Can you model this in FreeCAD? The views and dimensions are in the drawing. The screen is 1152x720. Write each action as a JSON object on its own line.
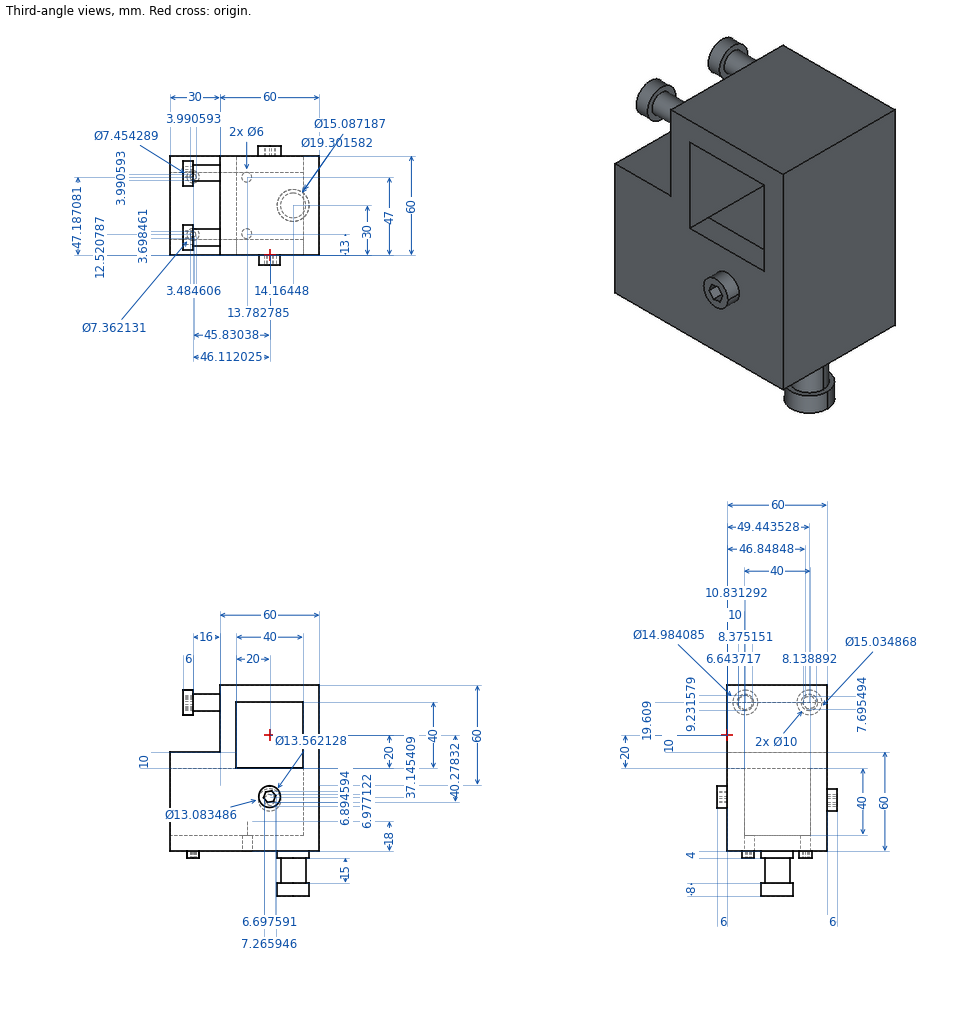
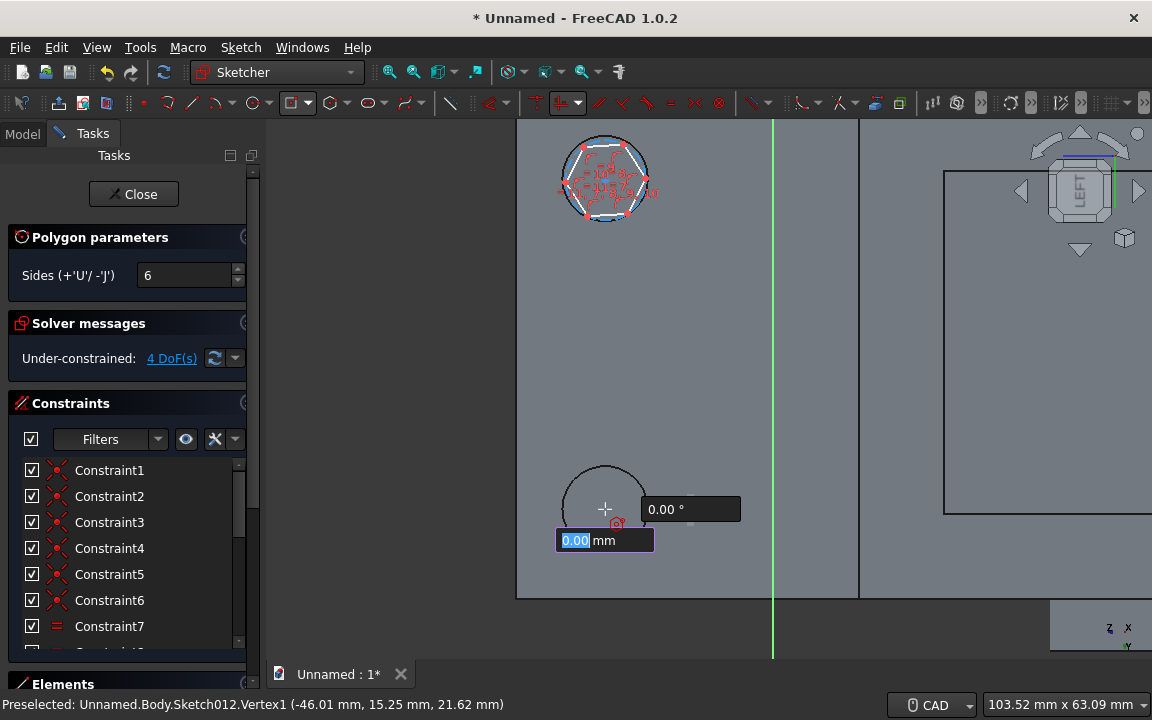
{"action": "left_click", "coordinate": [572, 522]}
{"action": "right_click", "coordinate": [572, 522]}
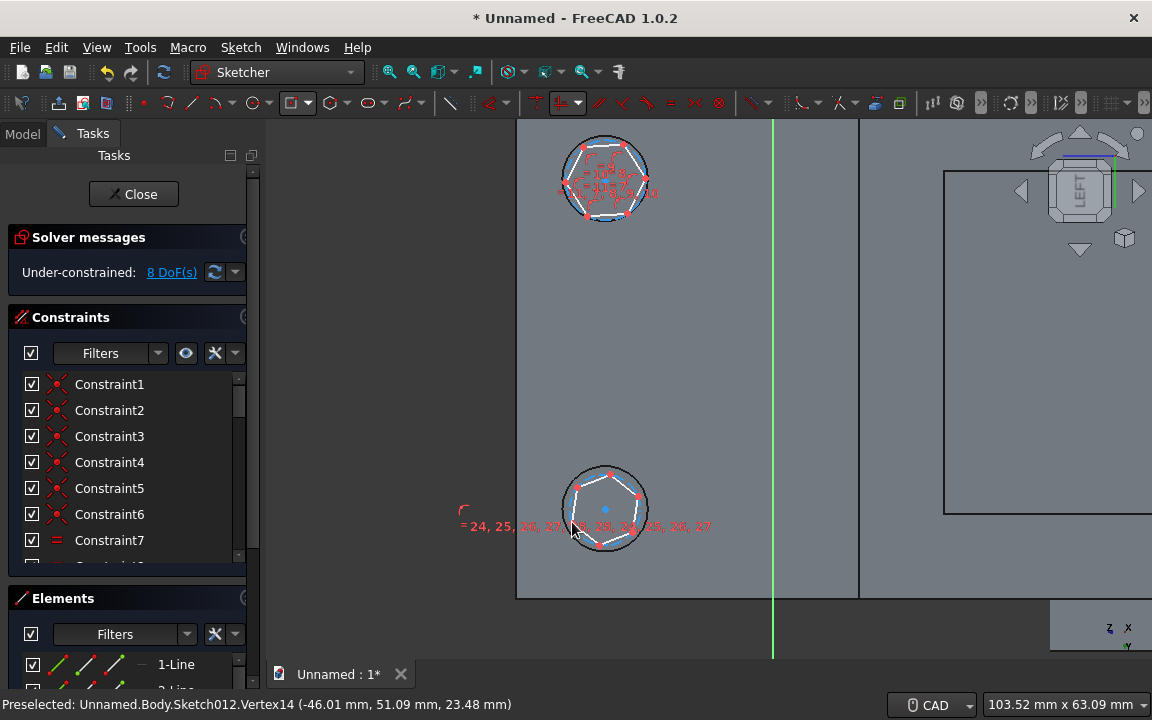
{"action": "left_click", "coordinate": [254, 104]}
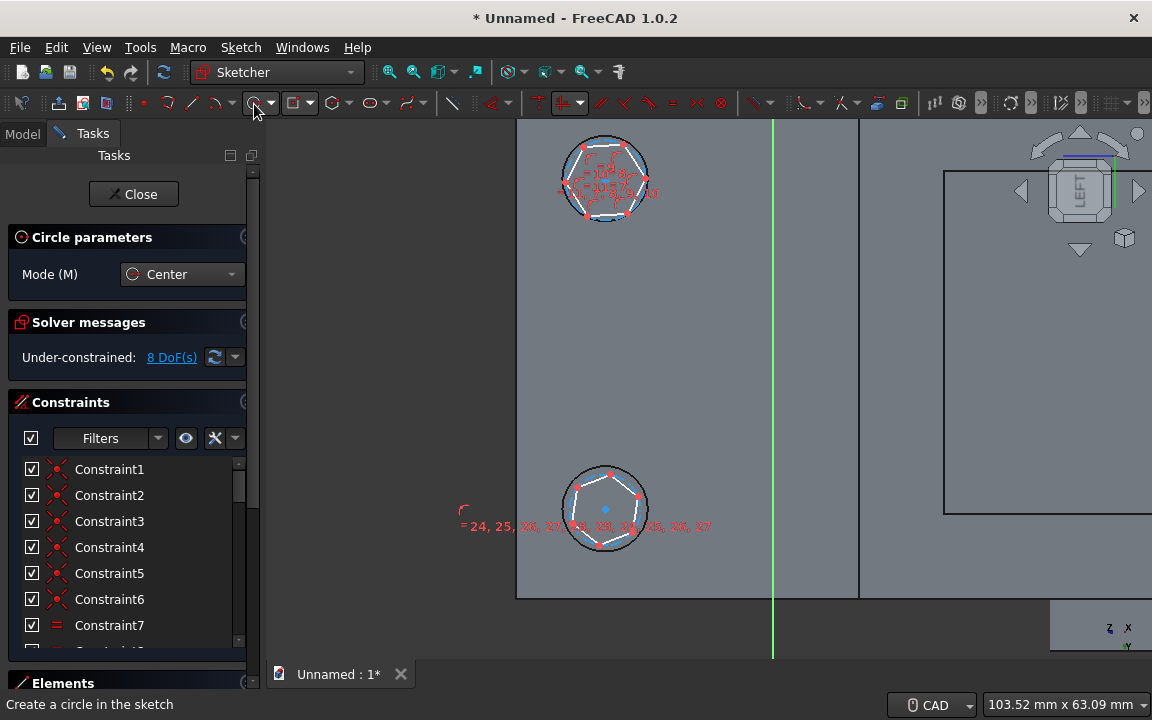
{"action": "left_click", "coordinate": [606, 180]}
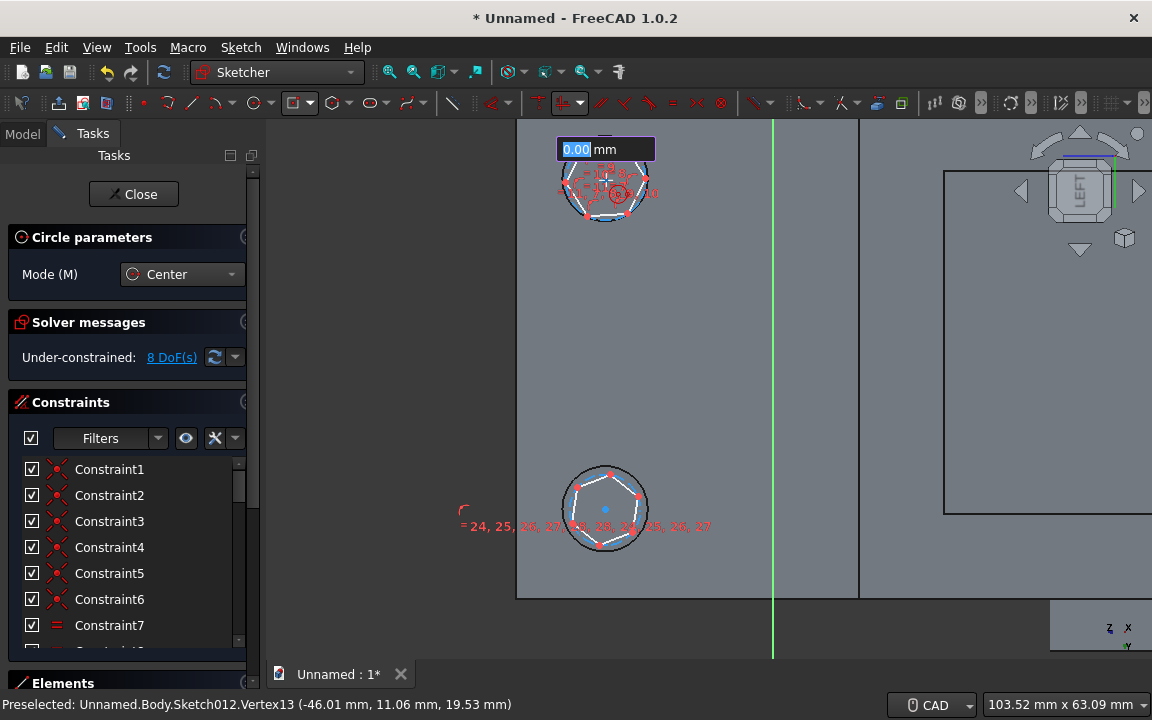
{"action": "scroll", "coordinate": [607, 510], "scroll_direction": "down", "scroll_amount": 2}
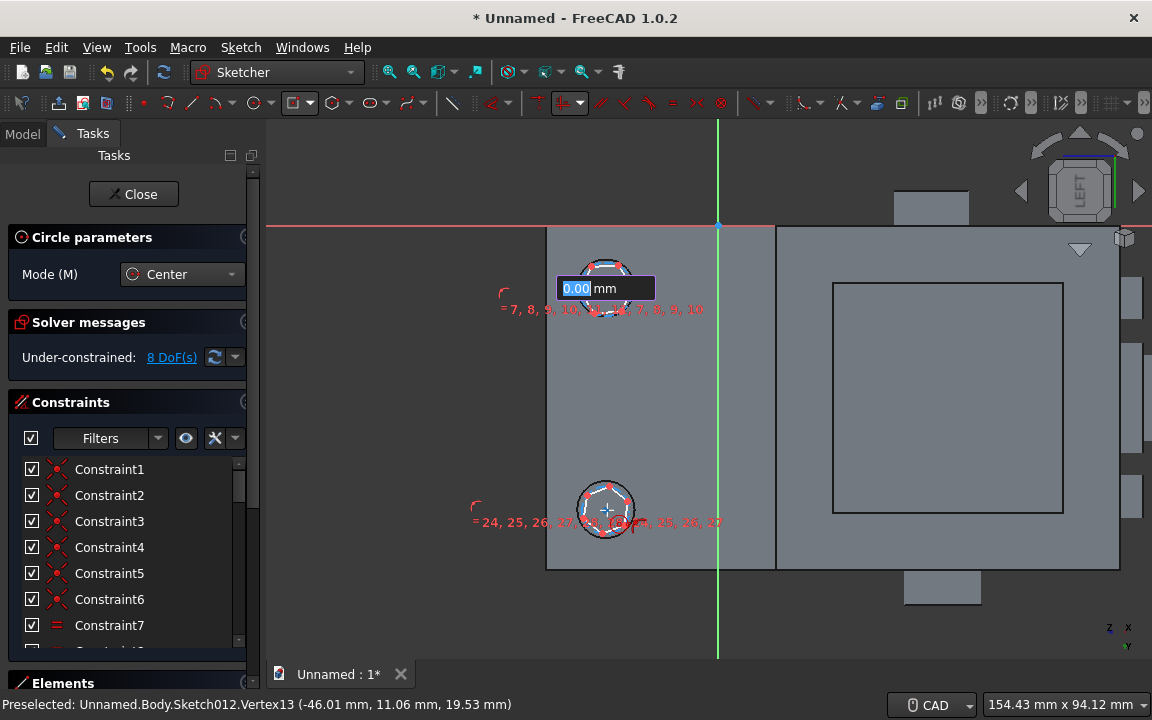
{"action": "left_click", "coordinate": [636, 258]}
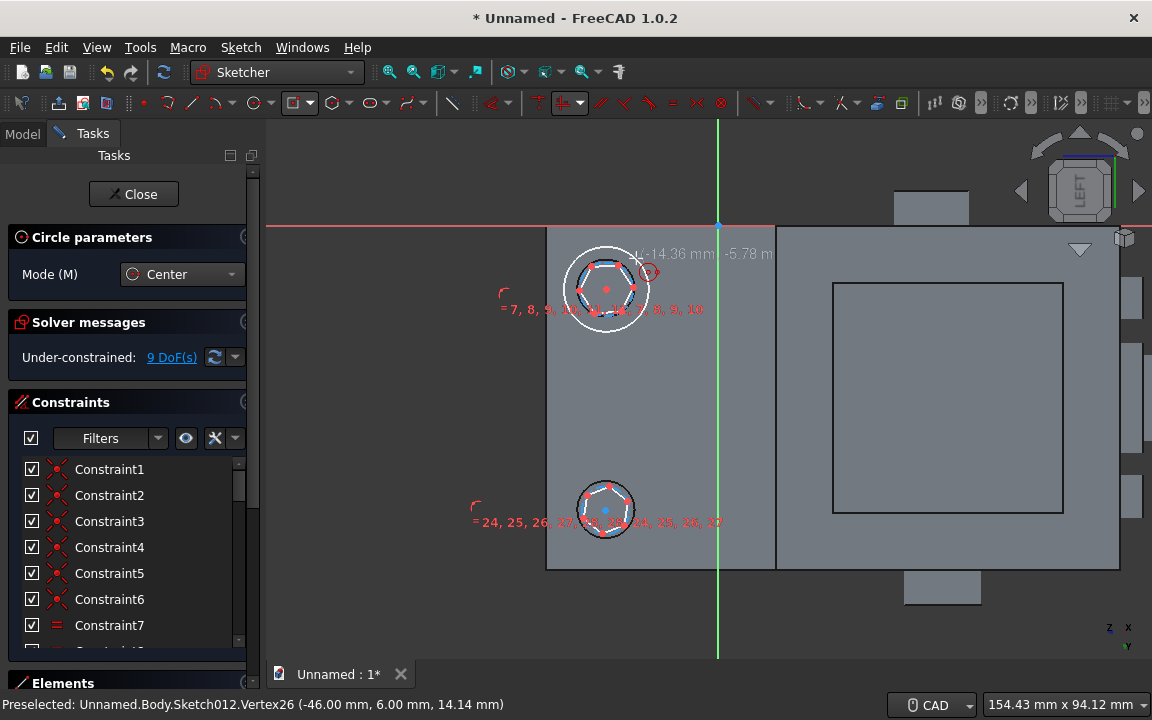
{"action": "left_click", "coordinate": [606, 510]}
{"action": "left_click", "coordinate": [636, 479]}
{"action": "key", "text": "Escape"}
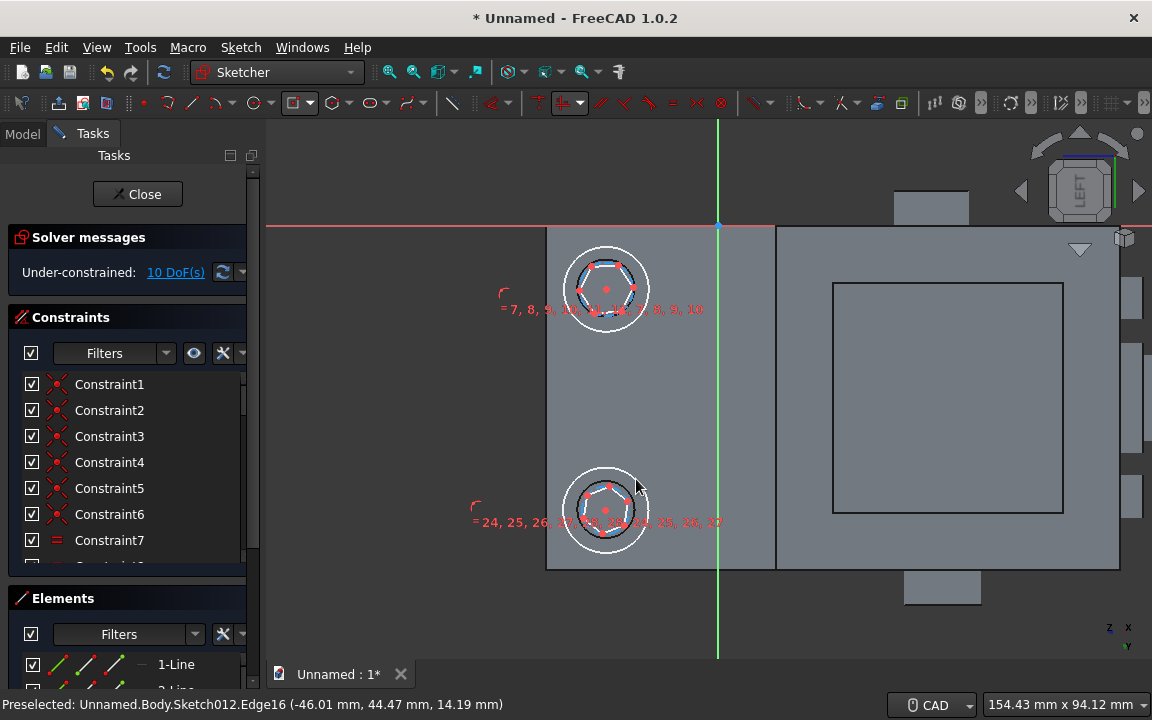
{"action": "left_click", "coordinate": [492, 104]}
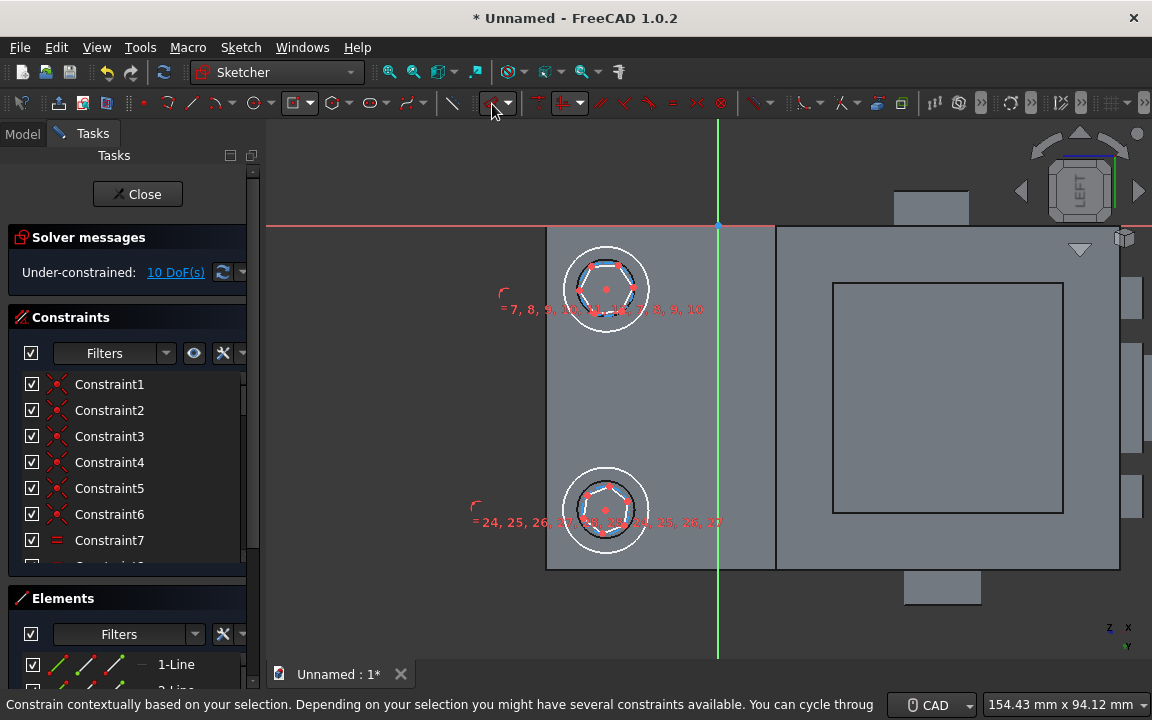
{"action": "left_click", "coordinate": [636, 259]}
{"action": "left_click", "coordinate": [678, 268]}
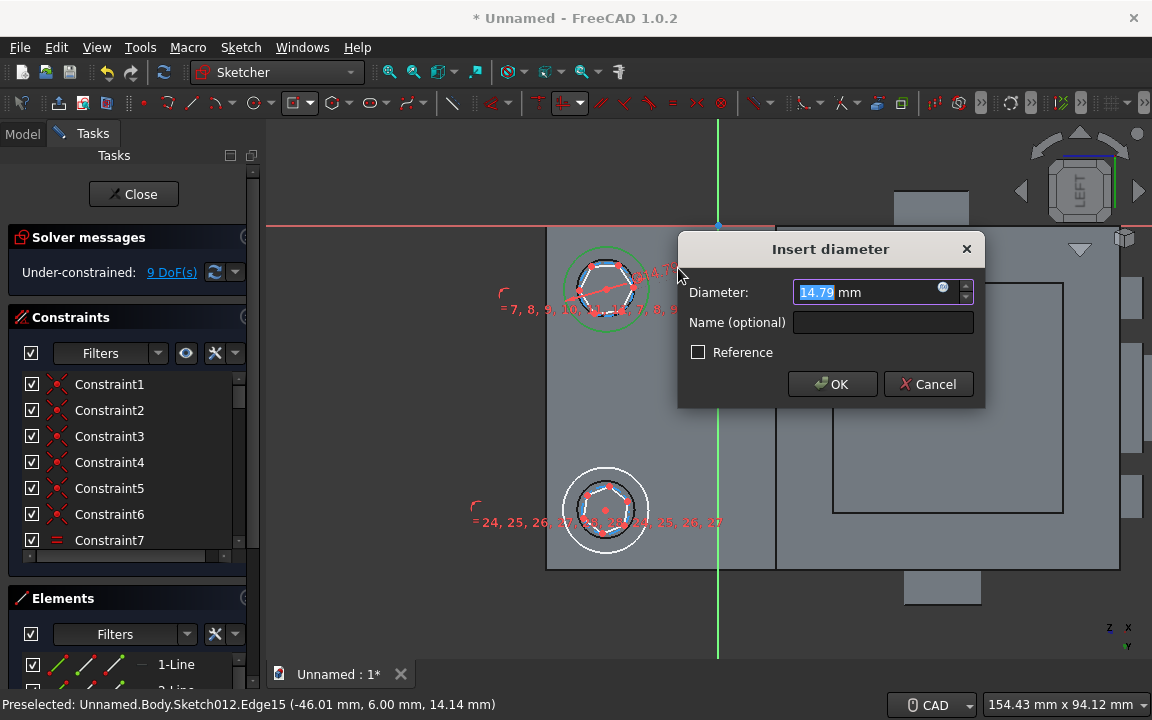
{"action": "type", "text": "14.984085"}
{"action": "key", "text": "Return"}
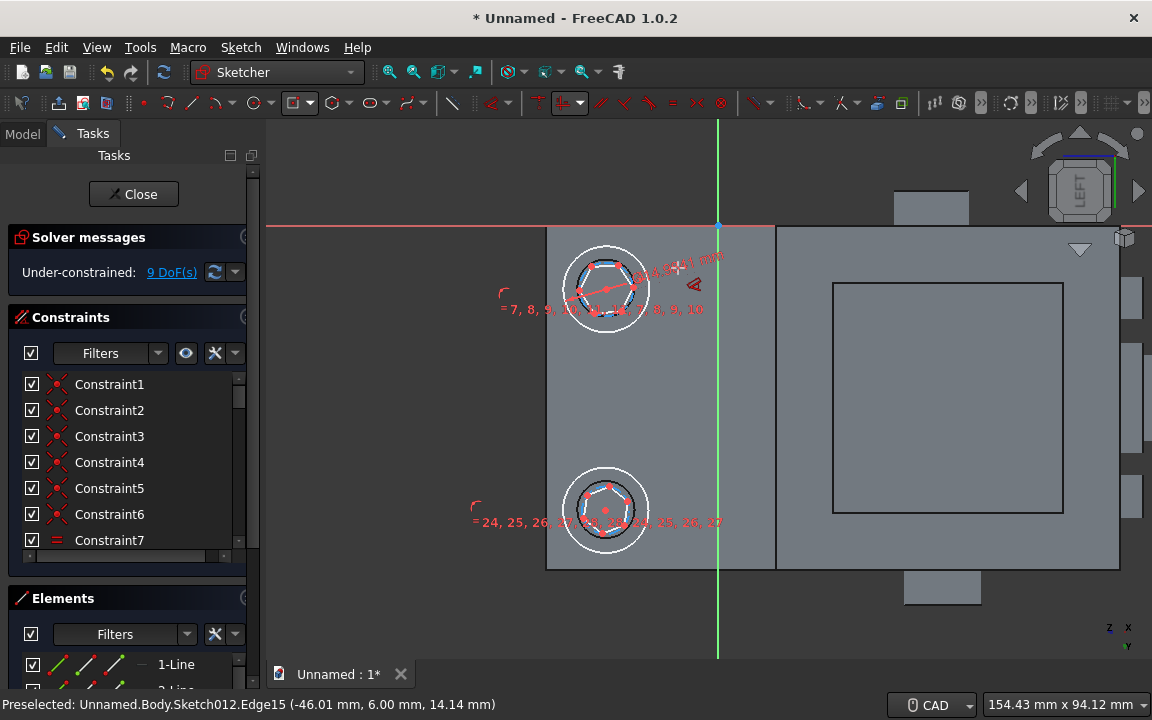
{"action": "left_click", "coordinate": [636, 480]}
{"action": "left_click", "coordinate": [659, 457]}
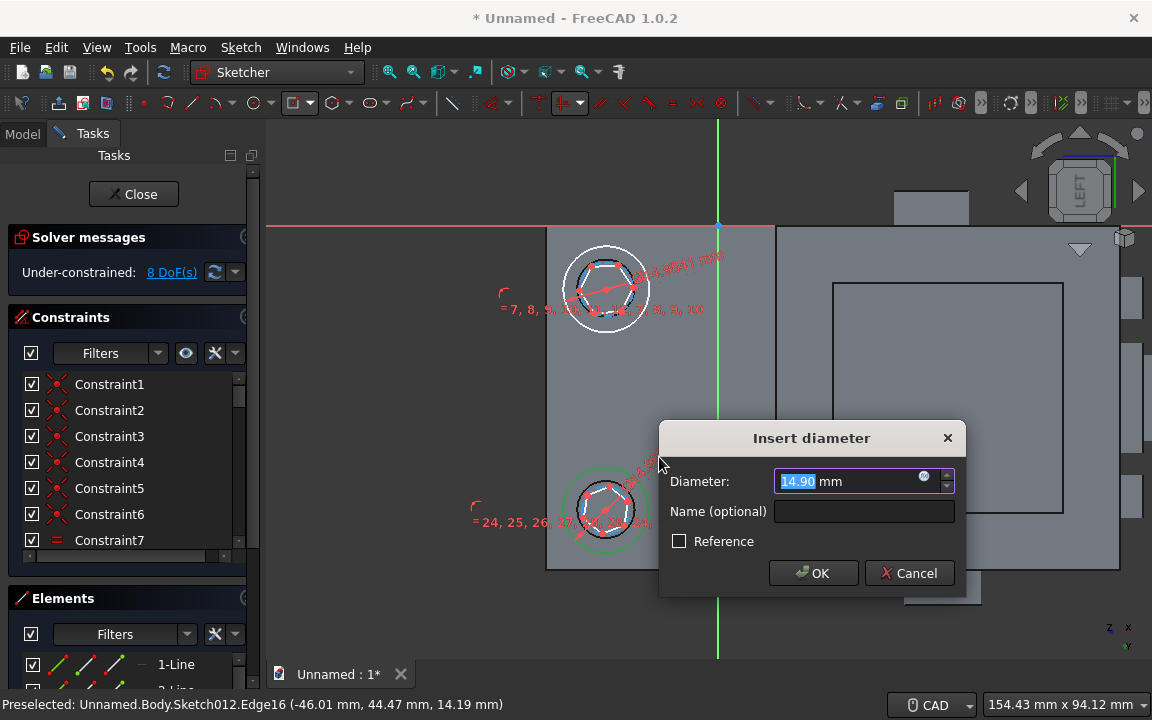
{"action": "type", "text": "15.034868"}
{"action": "key", "text": "Return"}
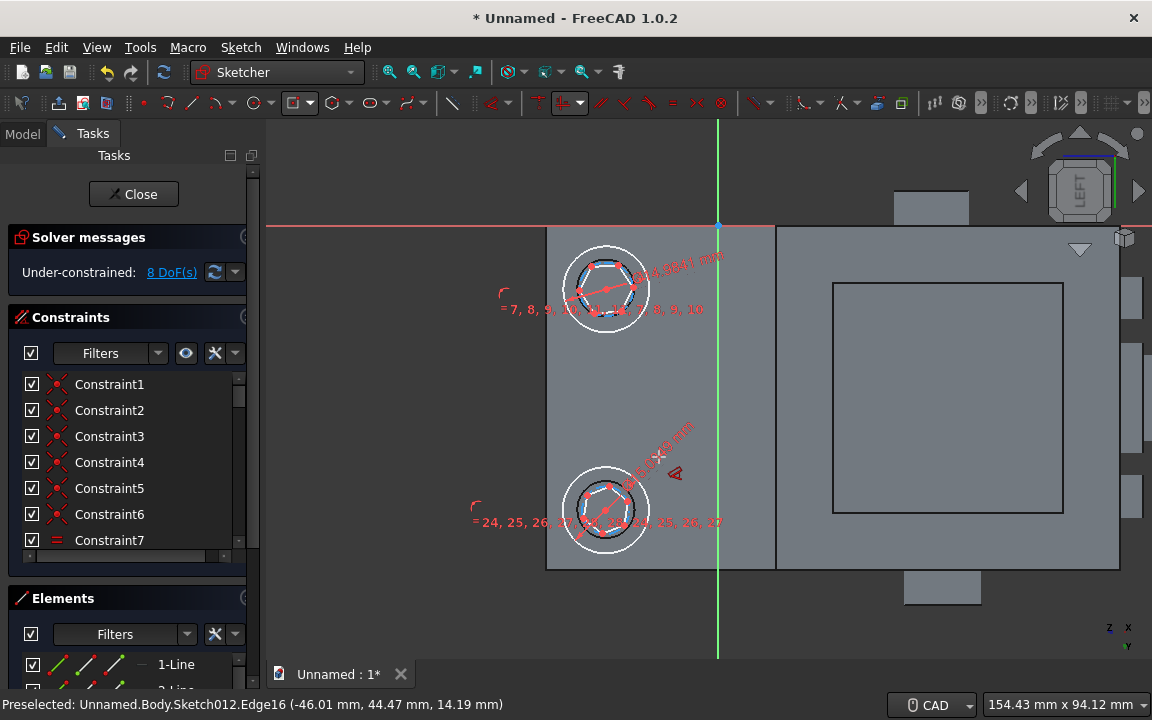
{"action": "left_click", "coordinate": [580, 291]}